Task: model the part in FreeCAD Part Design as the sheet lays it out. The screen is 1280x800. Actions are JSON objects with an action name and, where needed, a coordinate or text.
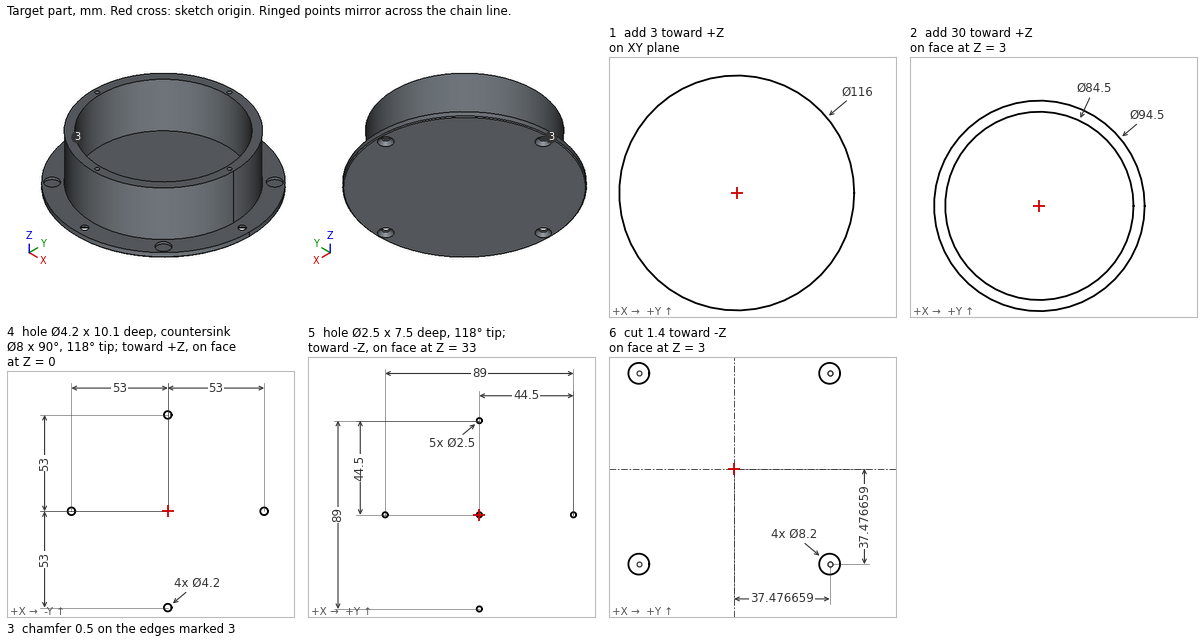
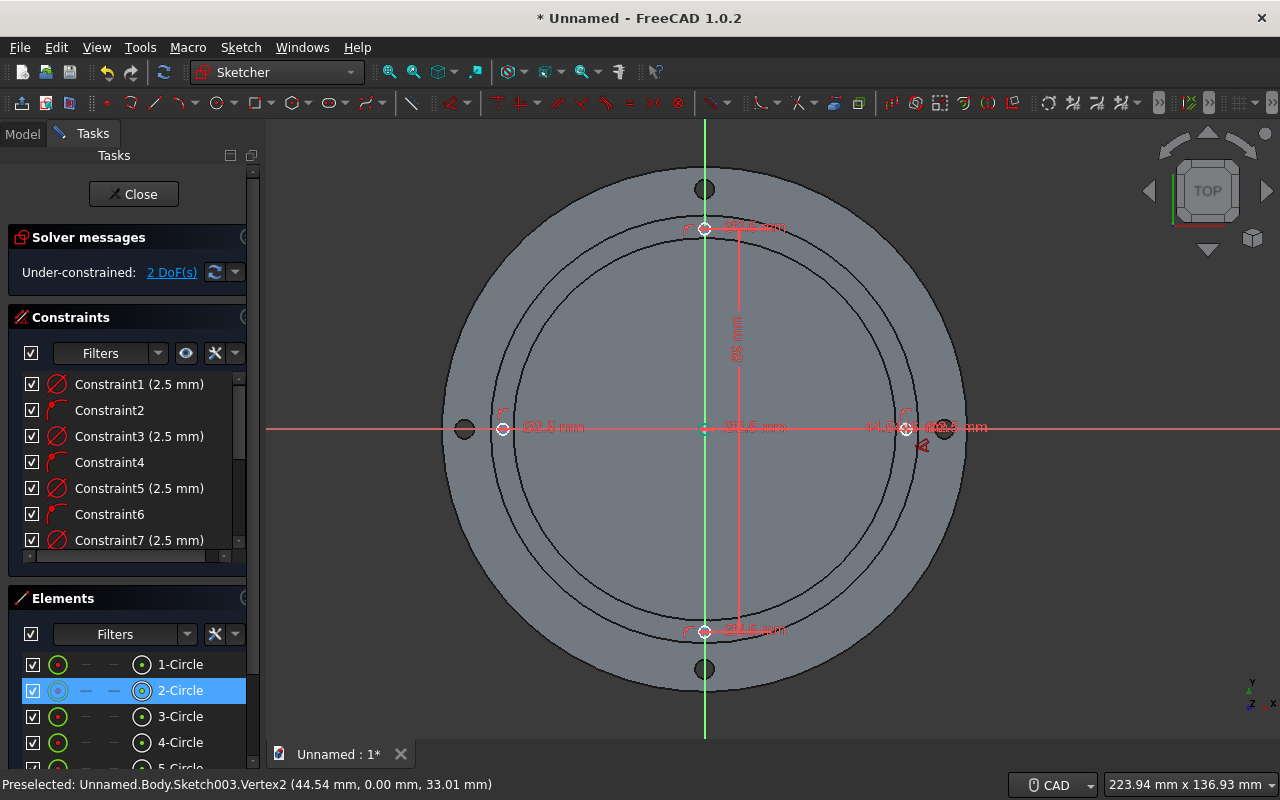
{"action": "left_click", "coordinate": [503, 429]}
{"action": "left_click", "coordinate": [612, 463]}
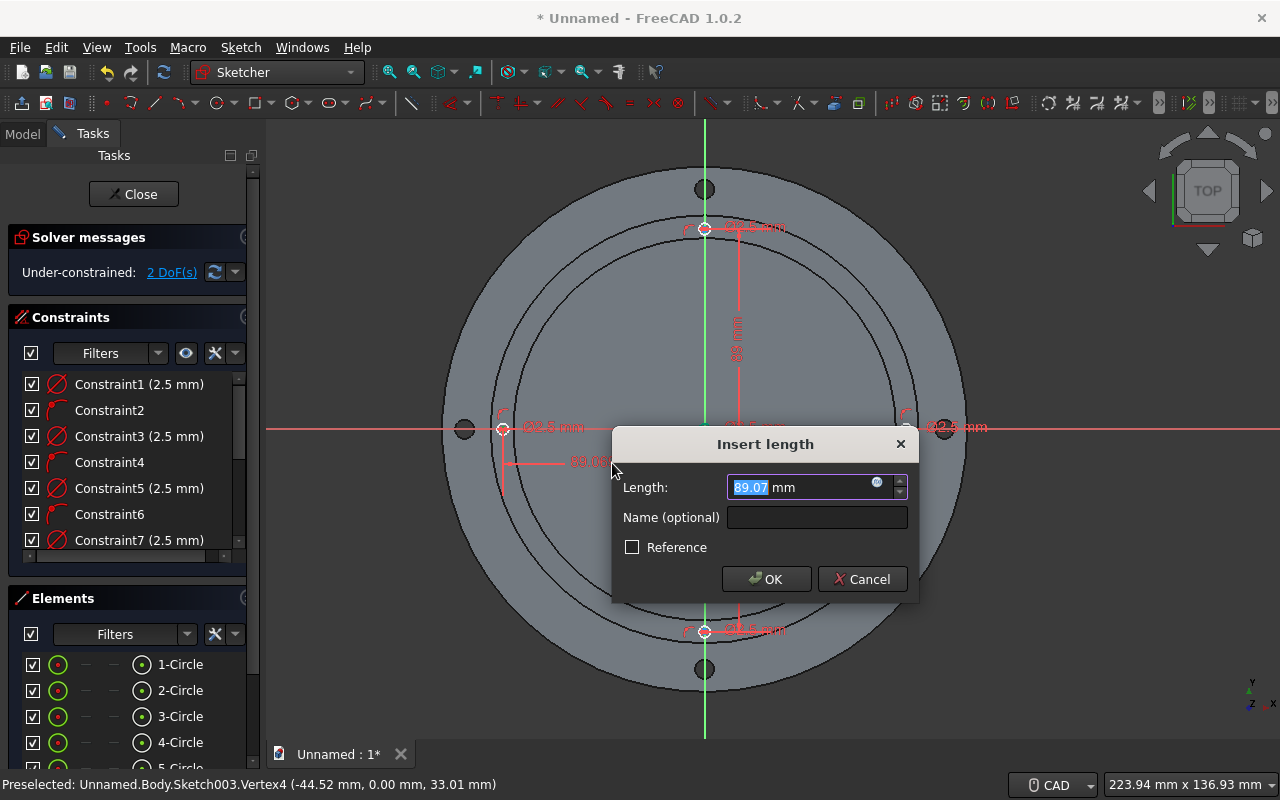
{"action": "type", "text": "89"}
{"action": "key", "text": "Return"}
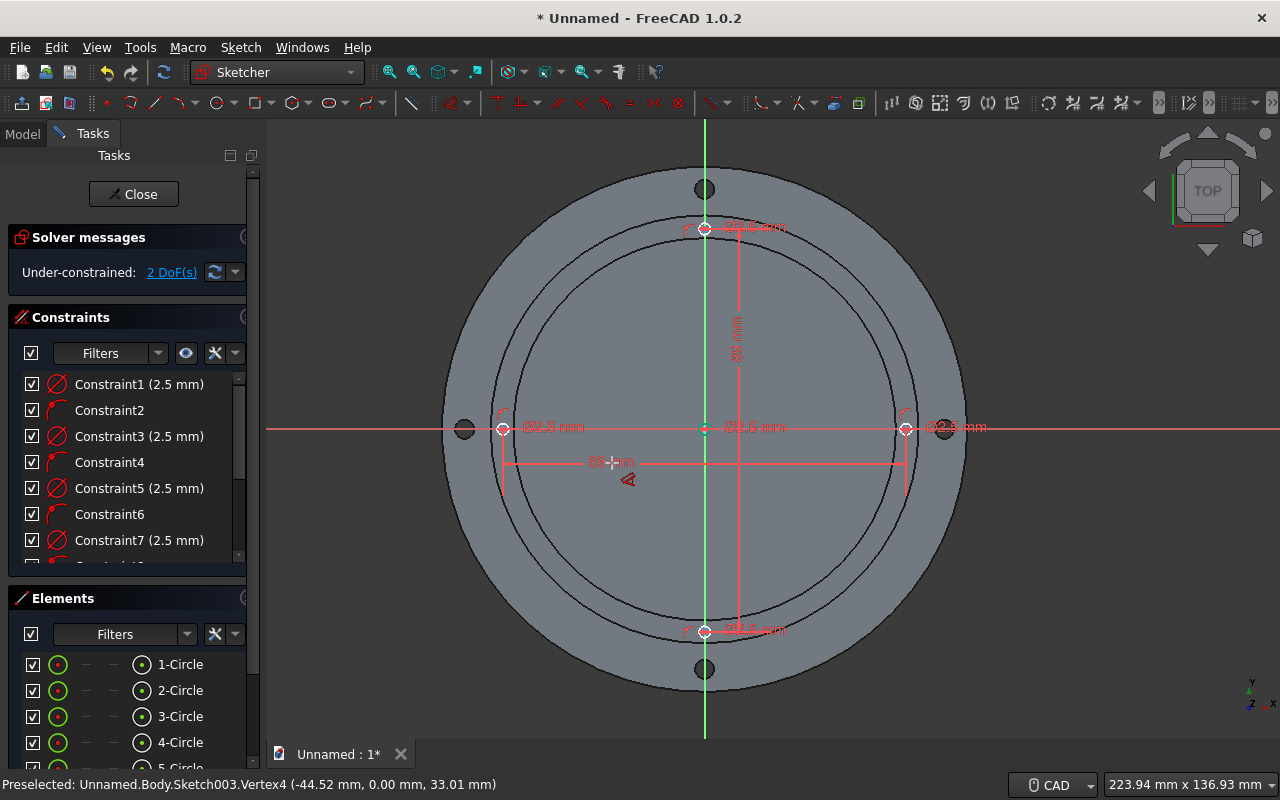
{"action": "left_click", "coordinate": [705, 229]}
{"action": "left_click", "coordinate": [739, 283]}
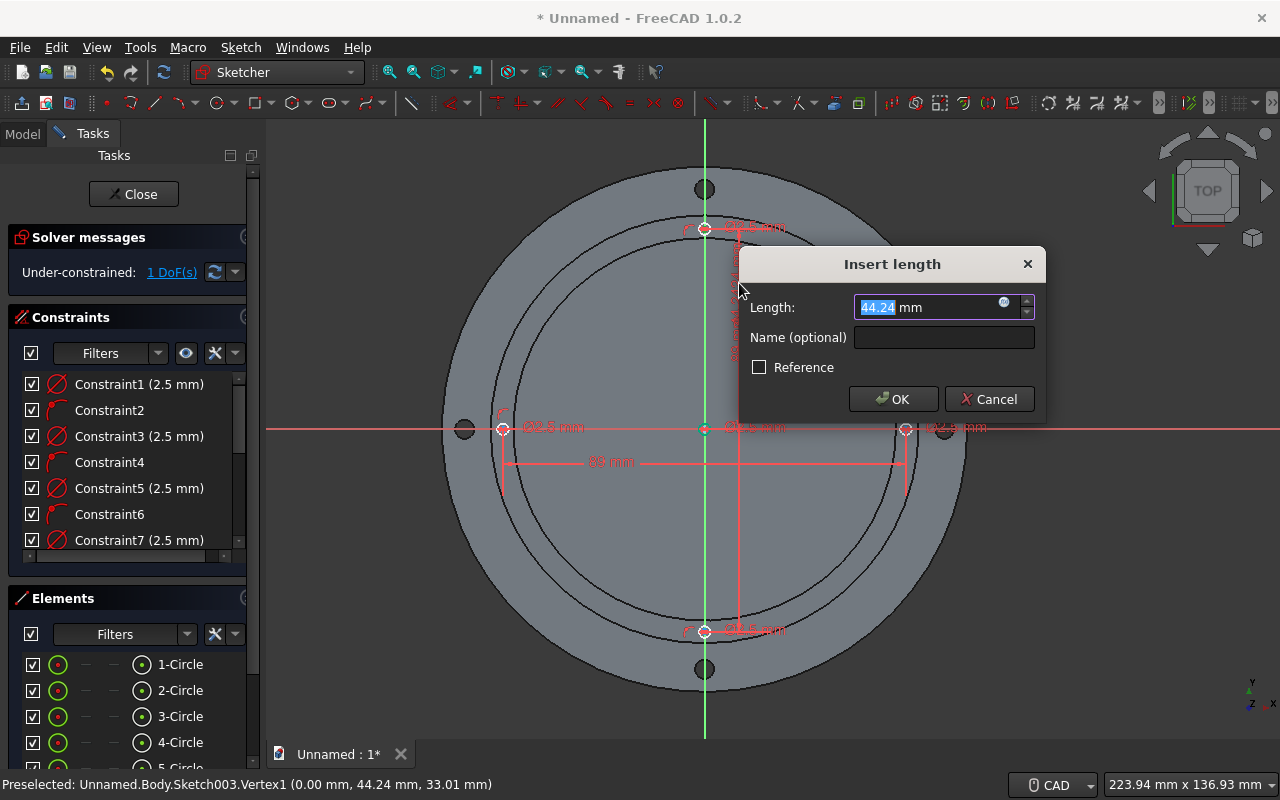
{"action": "type", "text": "44.5"}
{"action": "key", "text": "Return"}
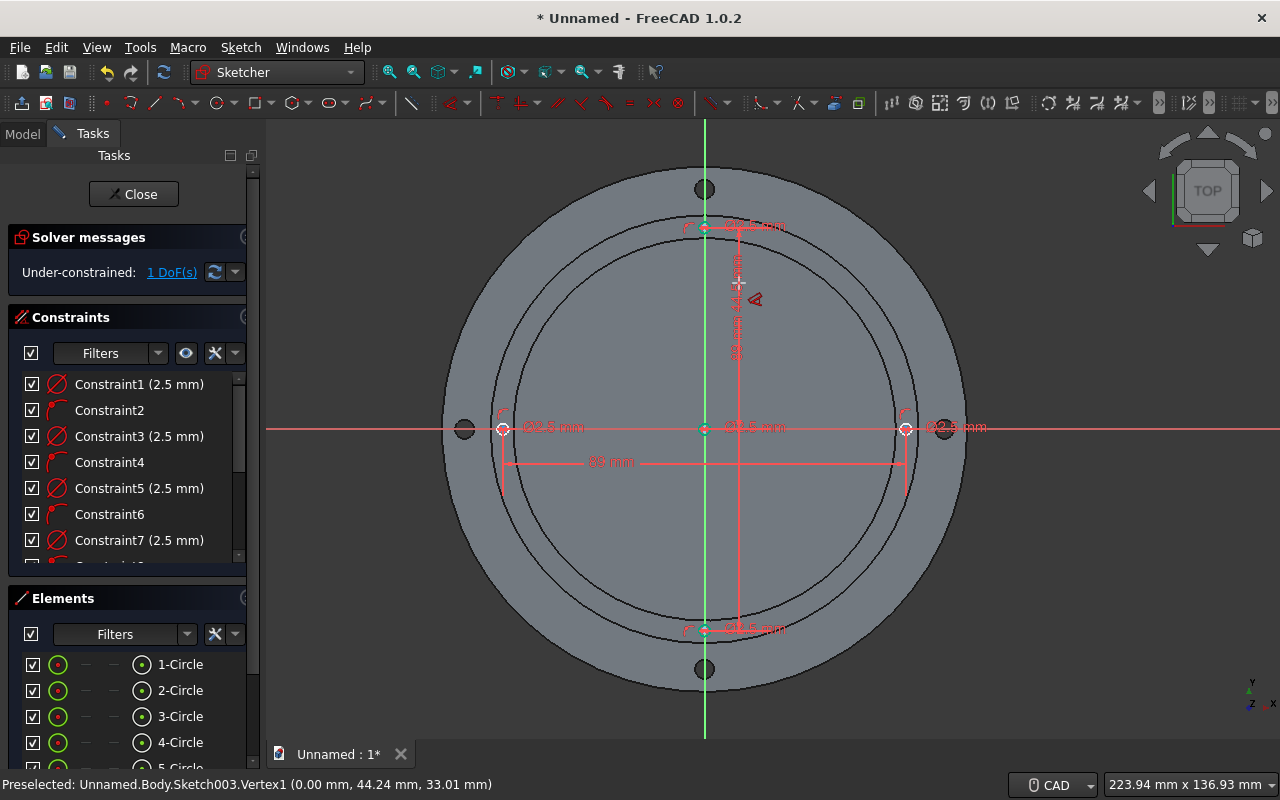
{"action": "left_click", "coordinate": [906, 429]}
{"action": "left_click", "coordinate": [805, 463]}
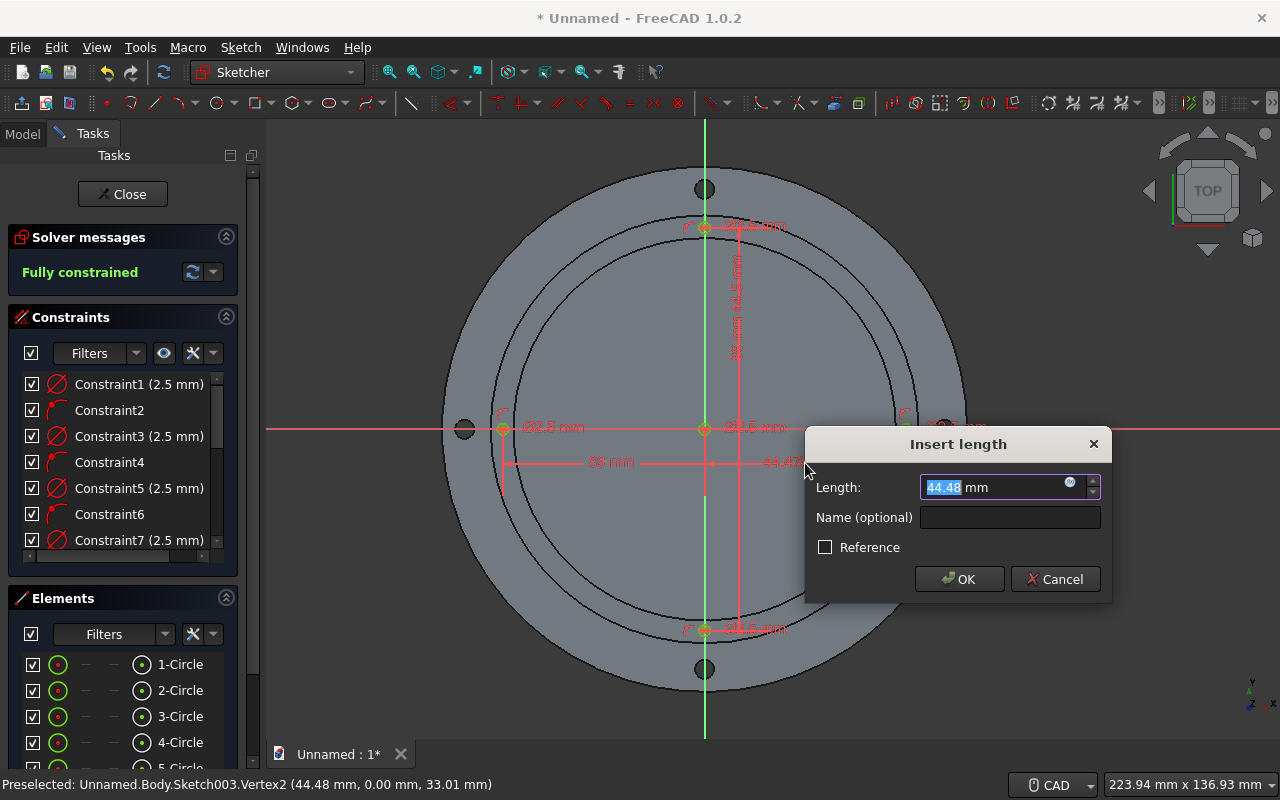
{"action": "type", "text": "44.5"}
{"action": "key", "text": "Return"}
{"action": "key", "text": "Escape"}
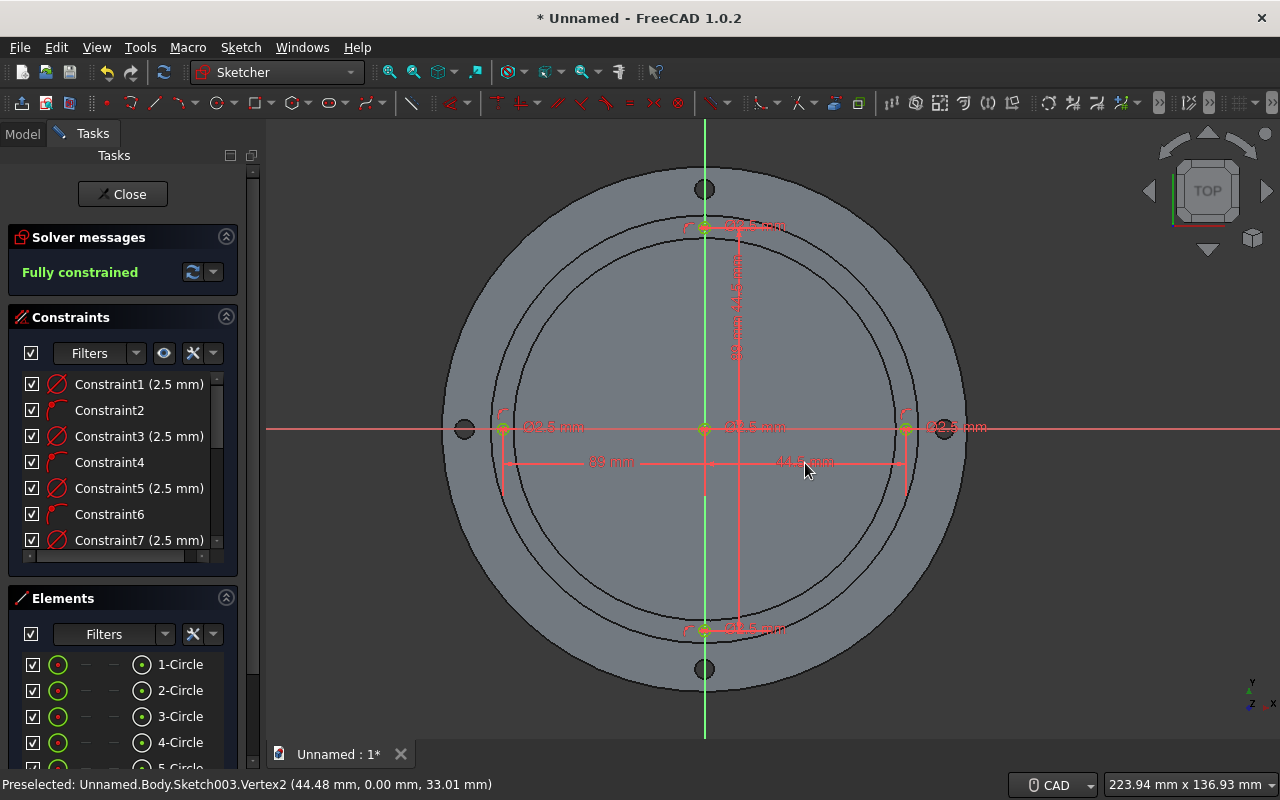
{"action": "left_click", "coordinate": [123, 194]}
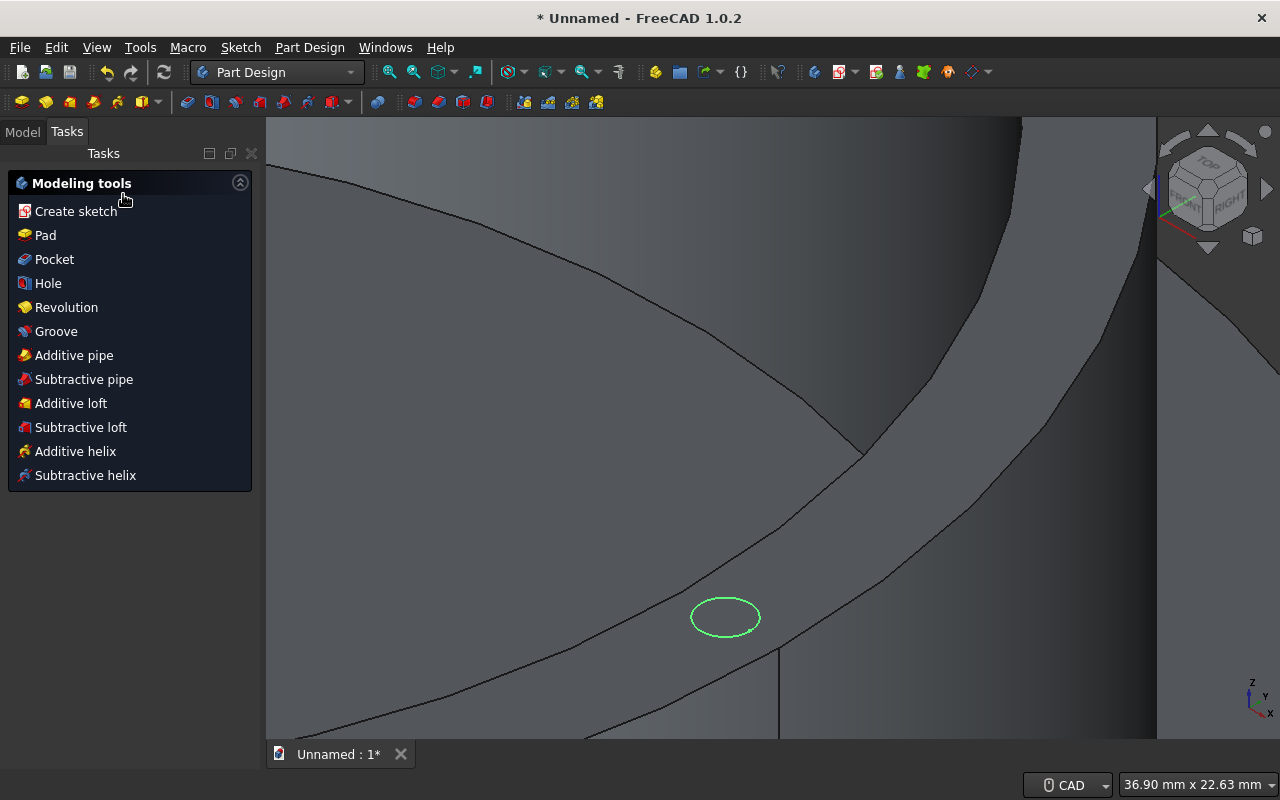
{"action": "left_click", "coordinate": [212, 102]}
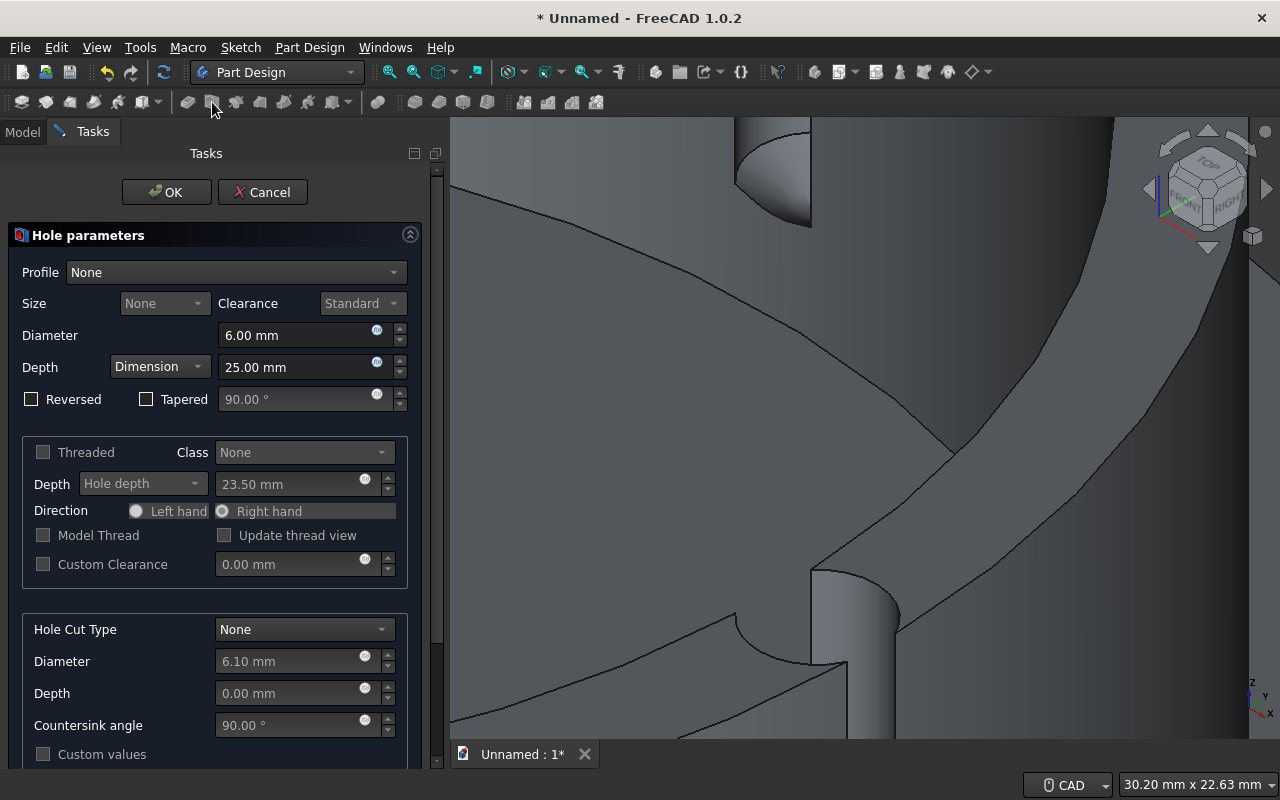
{"action": "triple_click", "coordinate": [305, 335]}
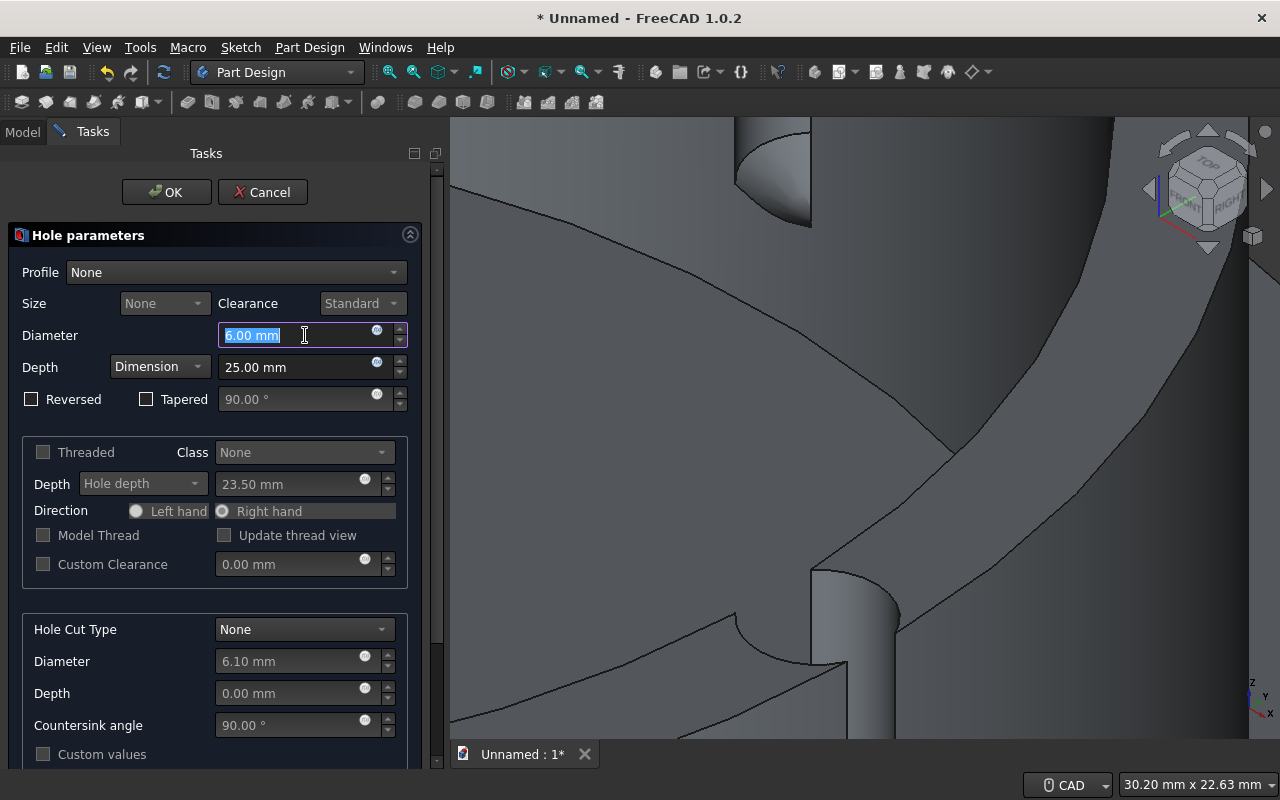
{"action": "type", "text": "2.5"}
{"action": "key", "text": "Tab"}